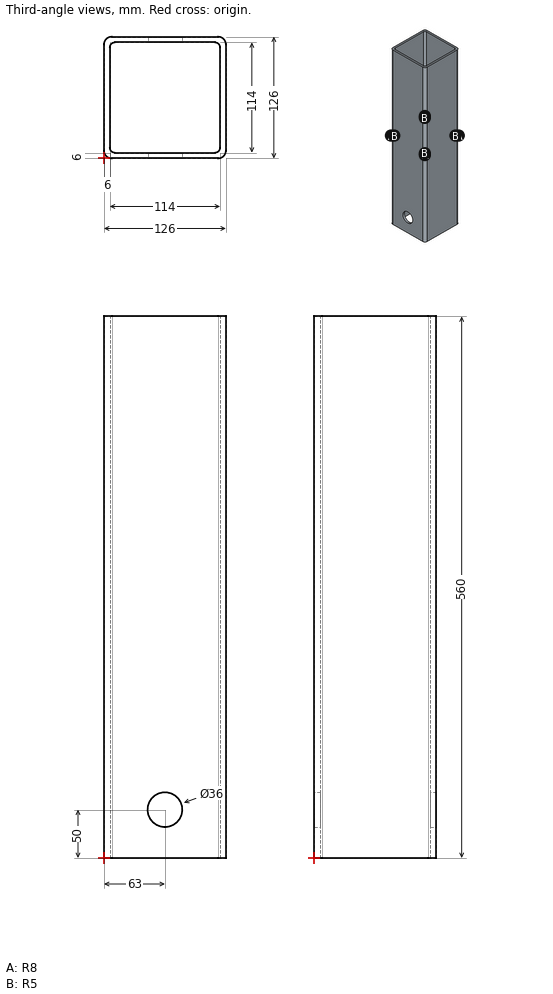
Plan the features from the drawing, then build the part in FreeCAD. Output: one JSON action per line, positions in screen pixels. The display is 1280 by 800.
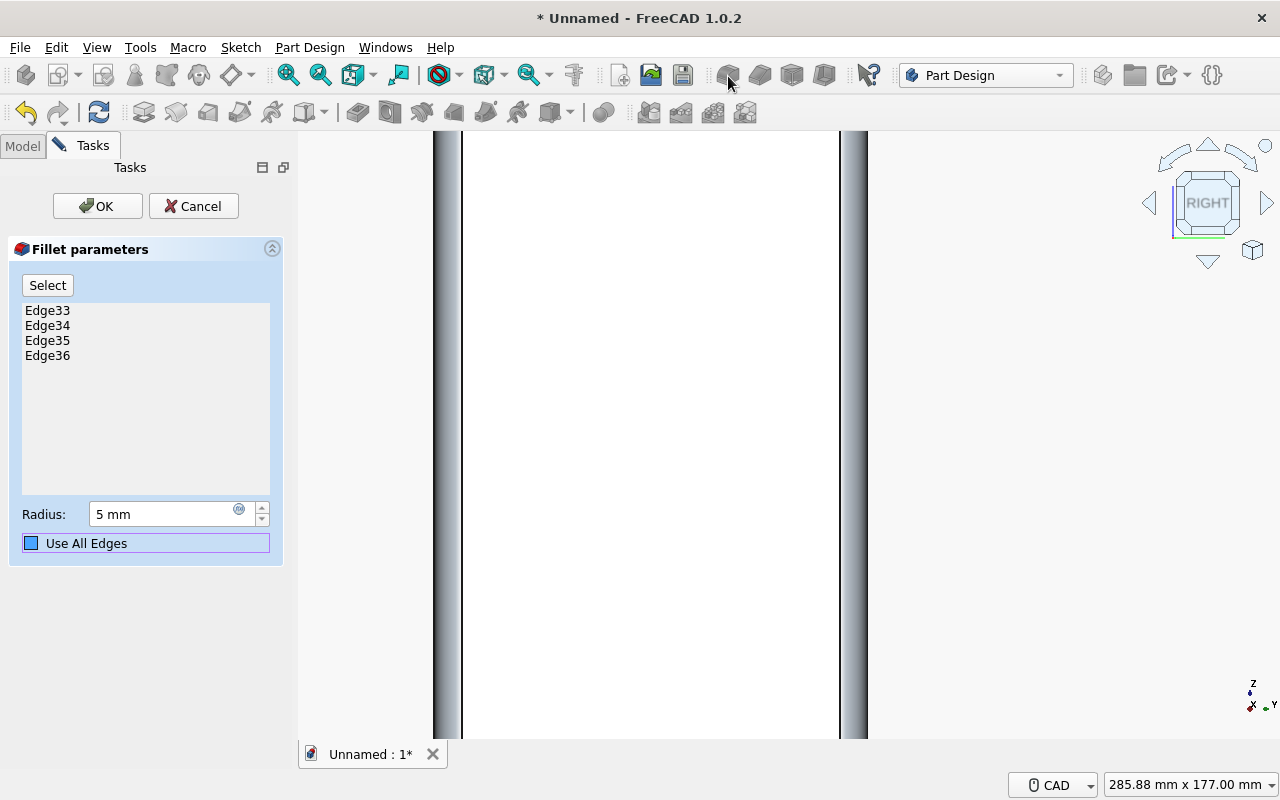
{"action": "left_click", "coordinate": [98, 206]}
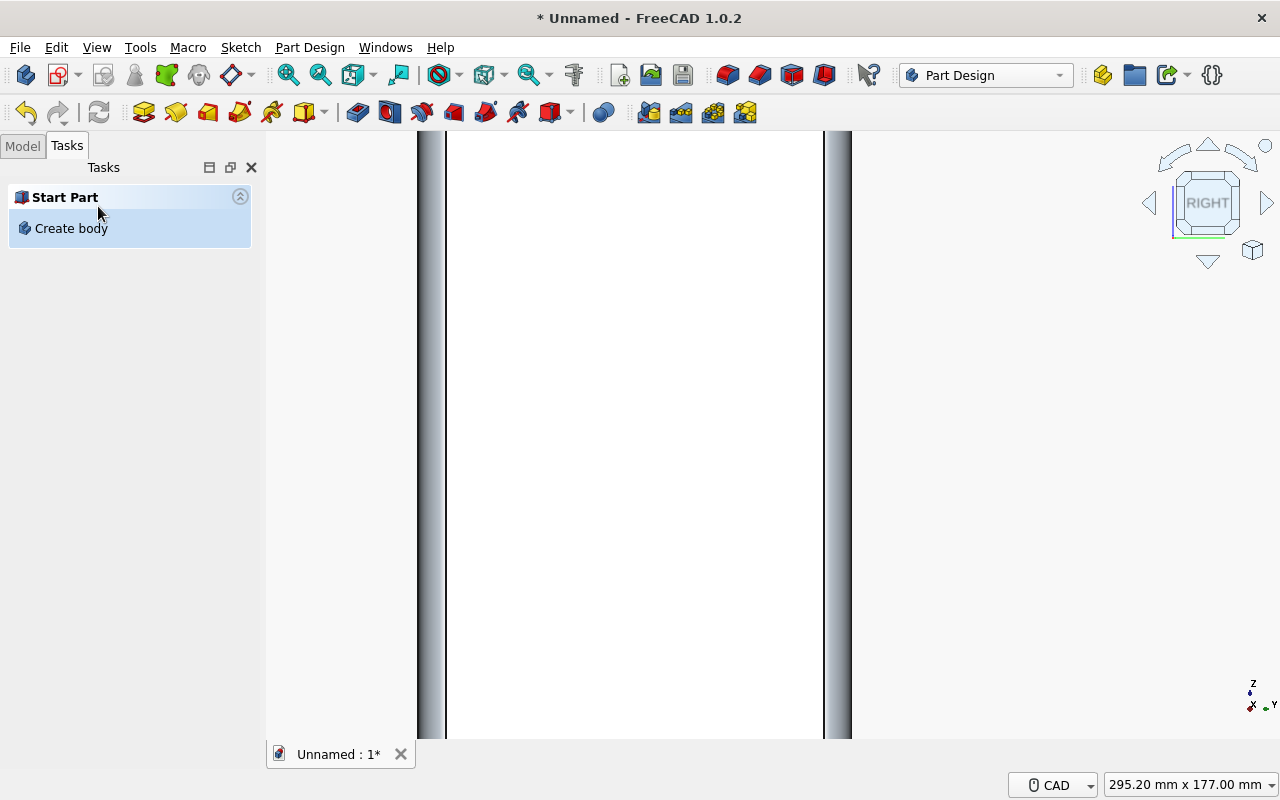
{"action": "left_click", "coordinate": [290, 76]}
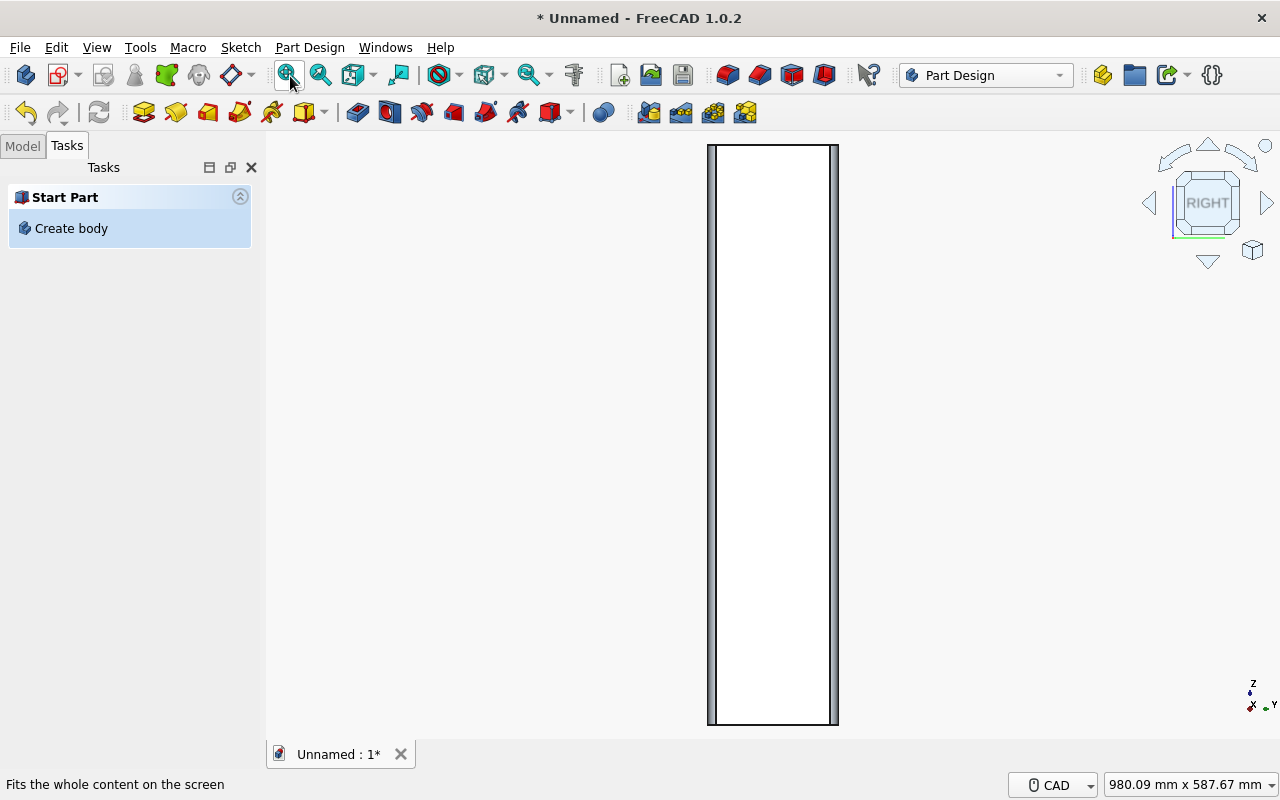
{"action": "left_click", "coordinate": [58, 76]}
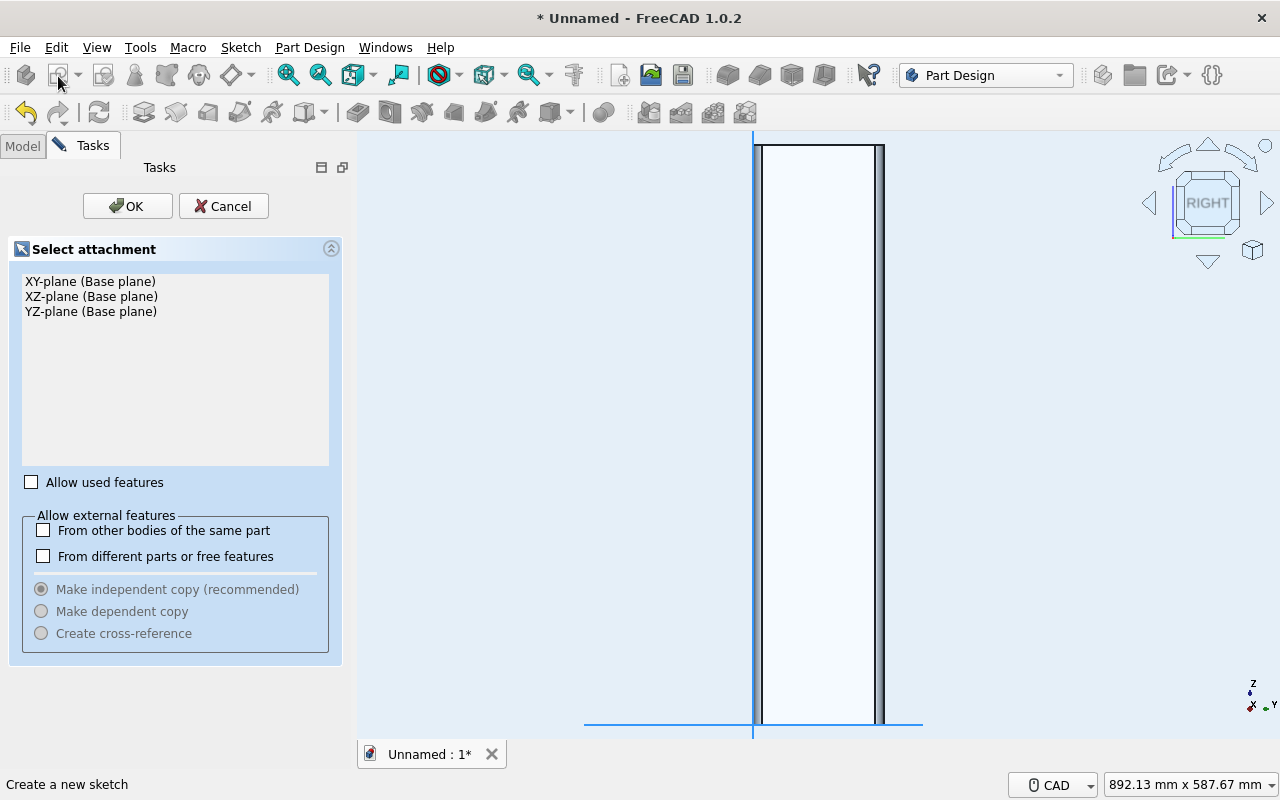
{"action": "left_click", "coordinate": [82, 296]}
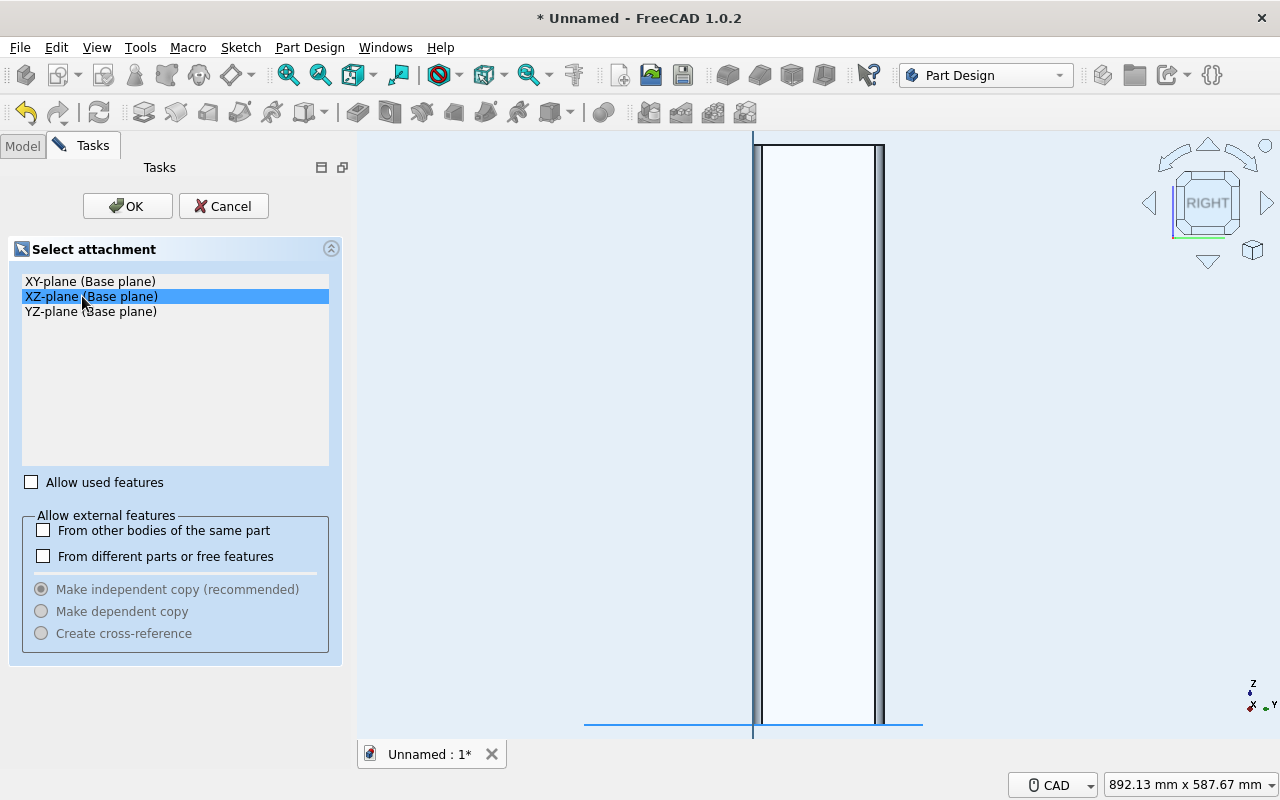
{"action": "left_click", "coordinate": [128, 206]}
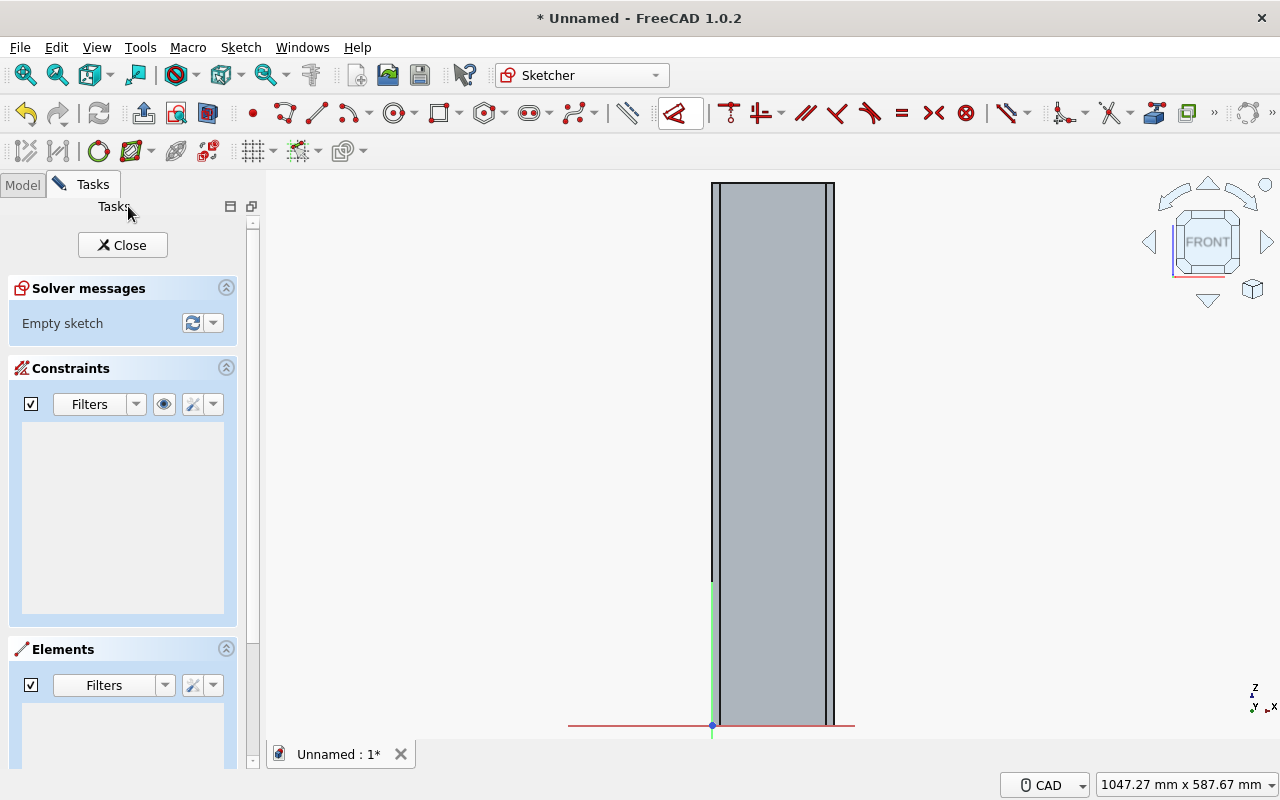
{"action": "scroll", "coordinate": [704, 454], "scroll_direction": "down", "scroll_amount": 5}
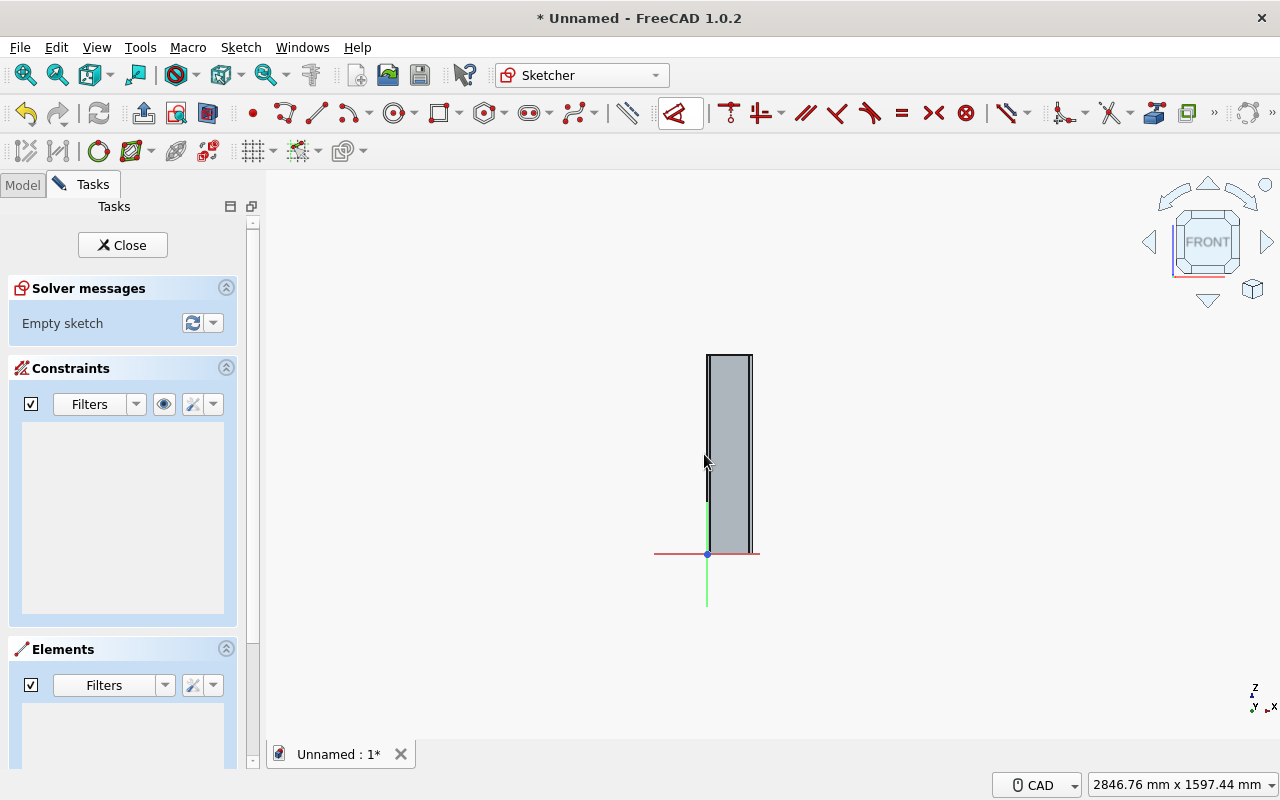
{"action": "scroll", "coordinate": [723, 548], "scroll_direction": "up", "scroll_amount": 14}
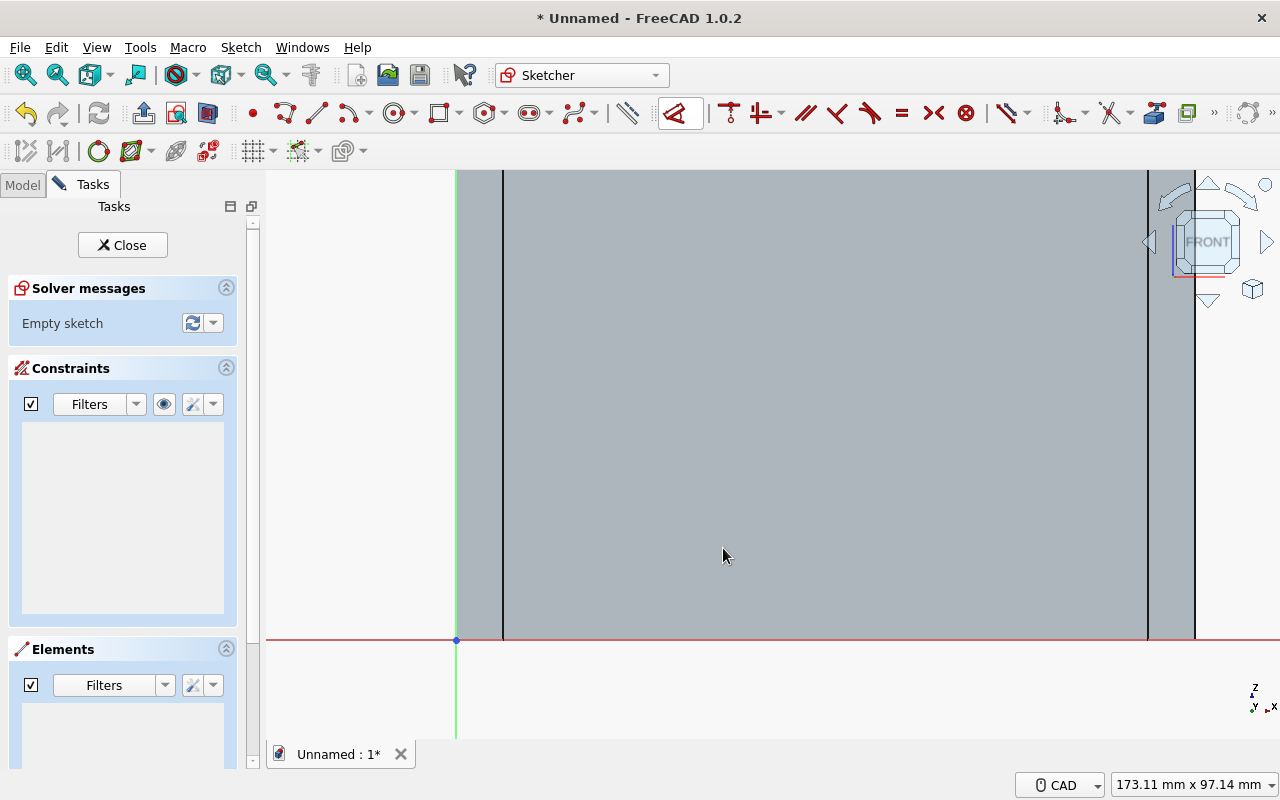
{"action": "left_click", "coordinate": [394, 114]}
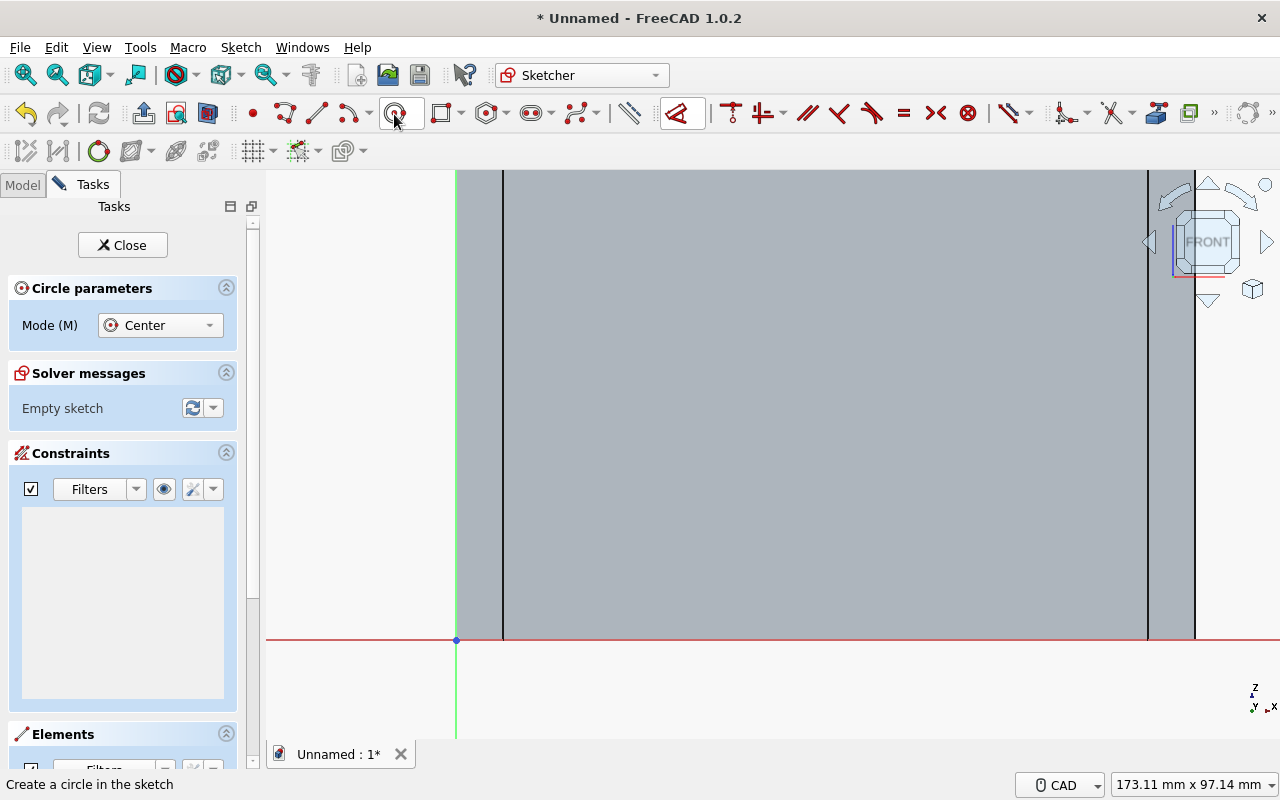
{"action": "left_click", "coordinate": [826, 347]}
{"action": "mouse_move", "coordinate": [900, 273]}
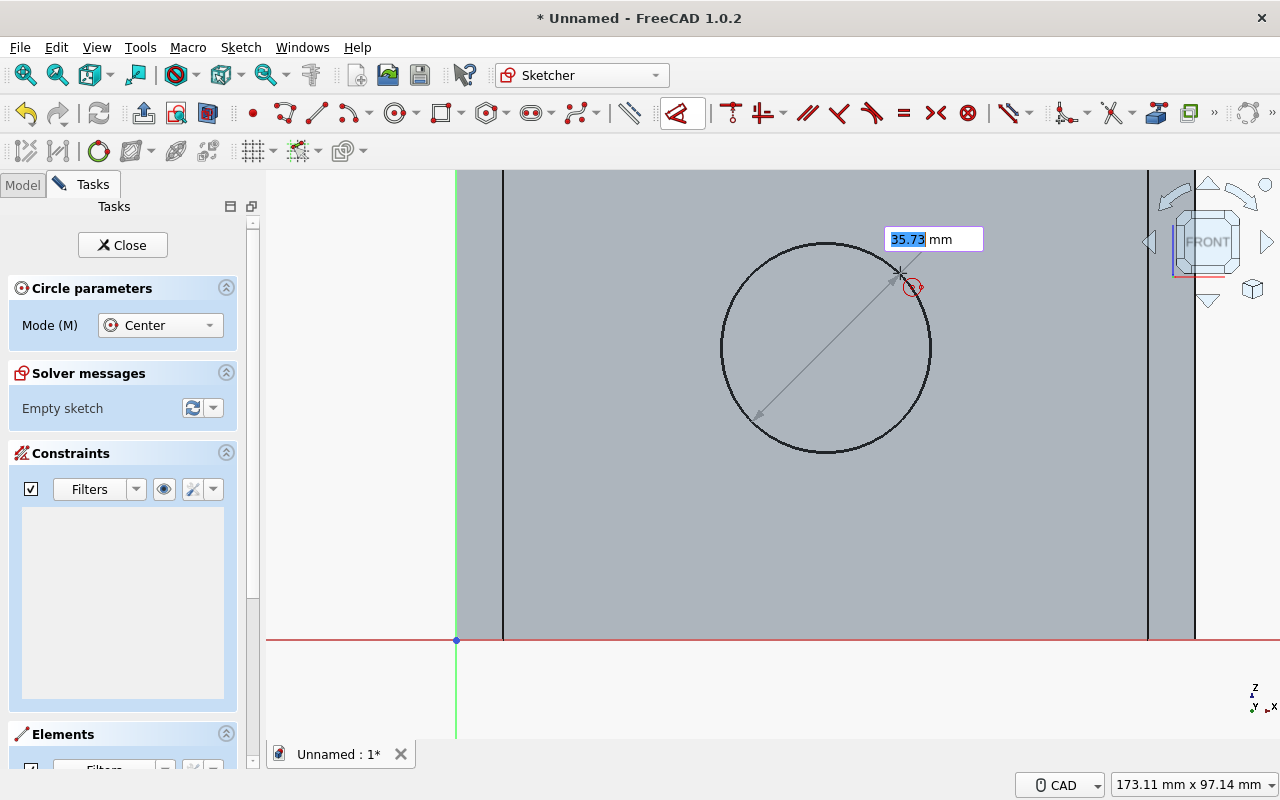
{"action": "type", "text": "36"}
{"action": "key", "text": "Return"}
{"action": "key", "text": "Escape"}